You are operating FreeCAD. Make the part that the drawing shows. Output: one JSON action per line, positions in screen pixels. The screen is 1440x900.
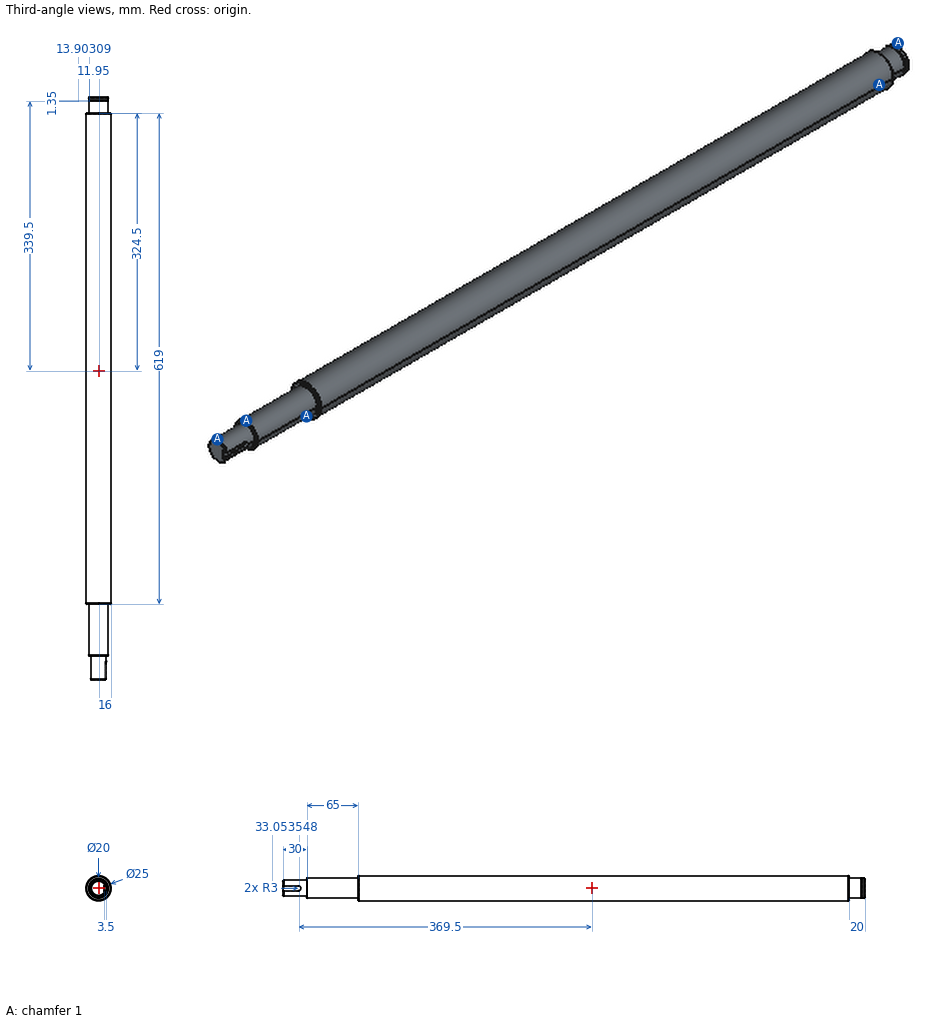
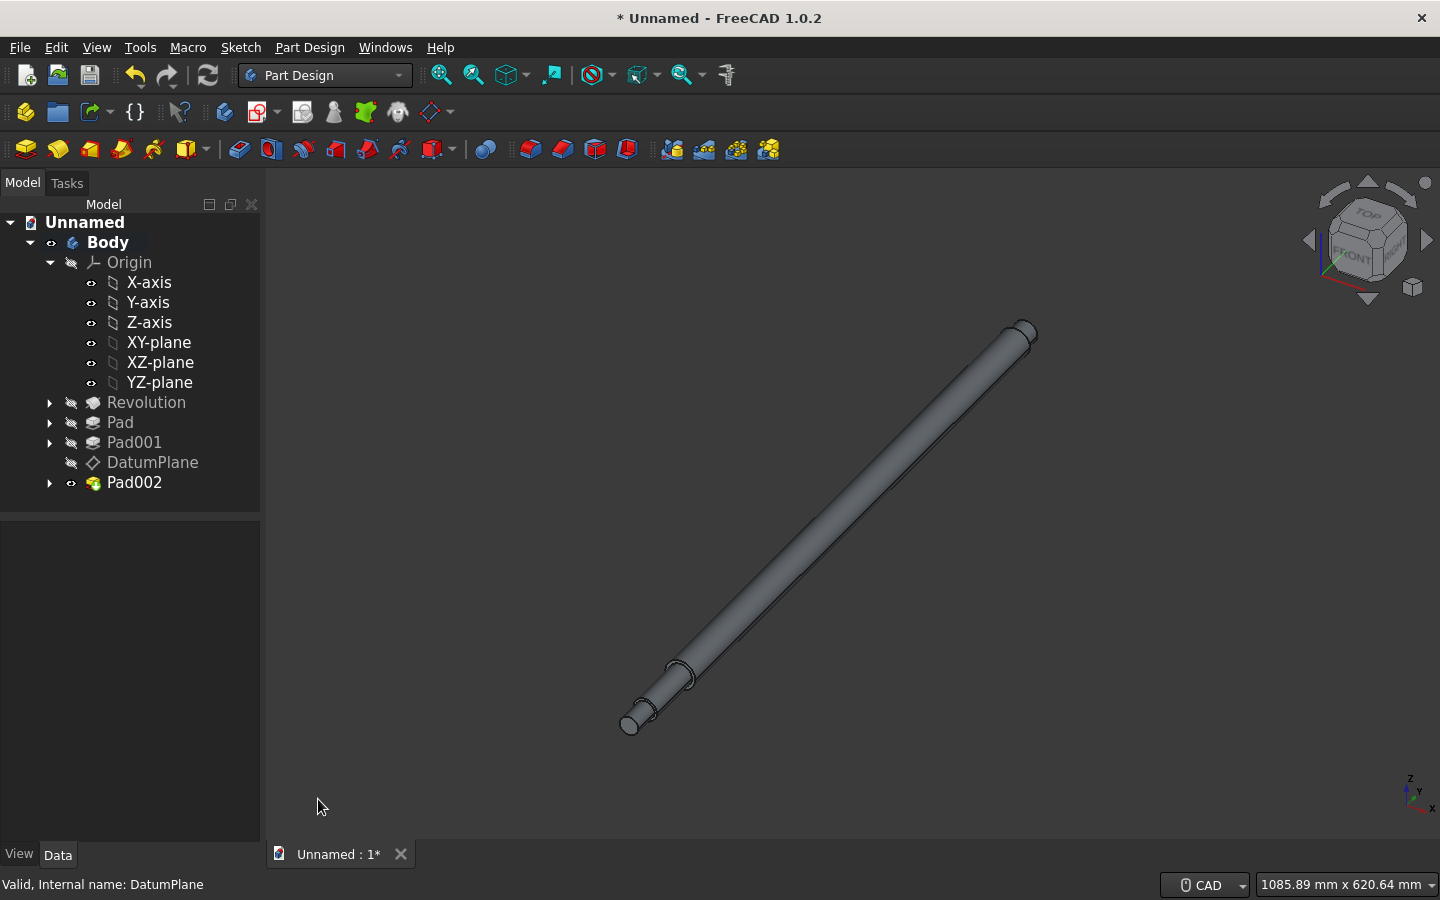
{"action": "left_click", "coordinate": [258, 112]}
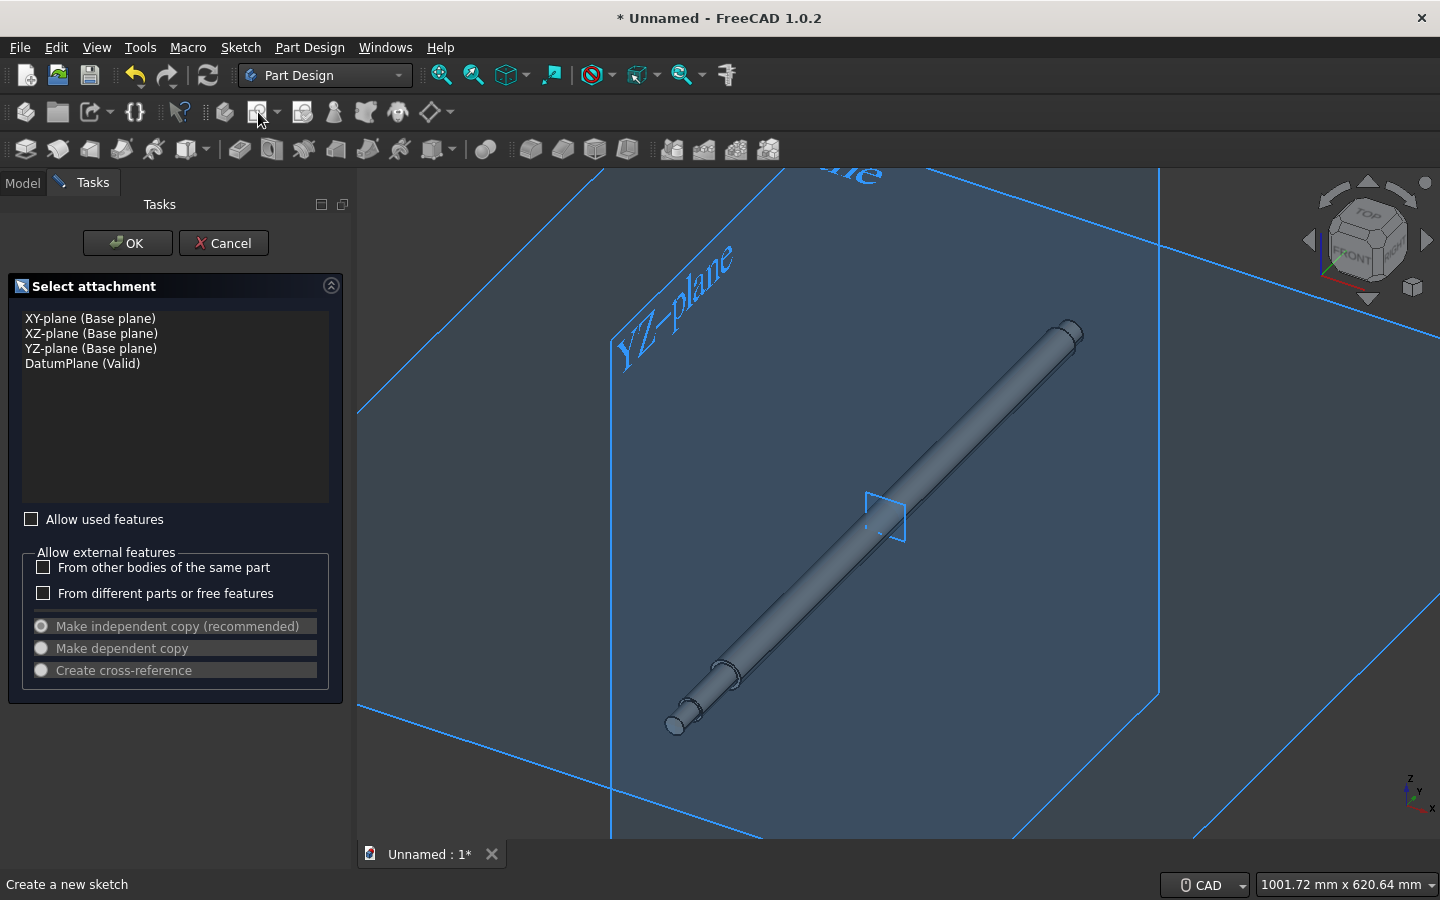
{"action": "left_click", "coordinate": [82, 318]}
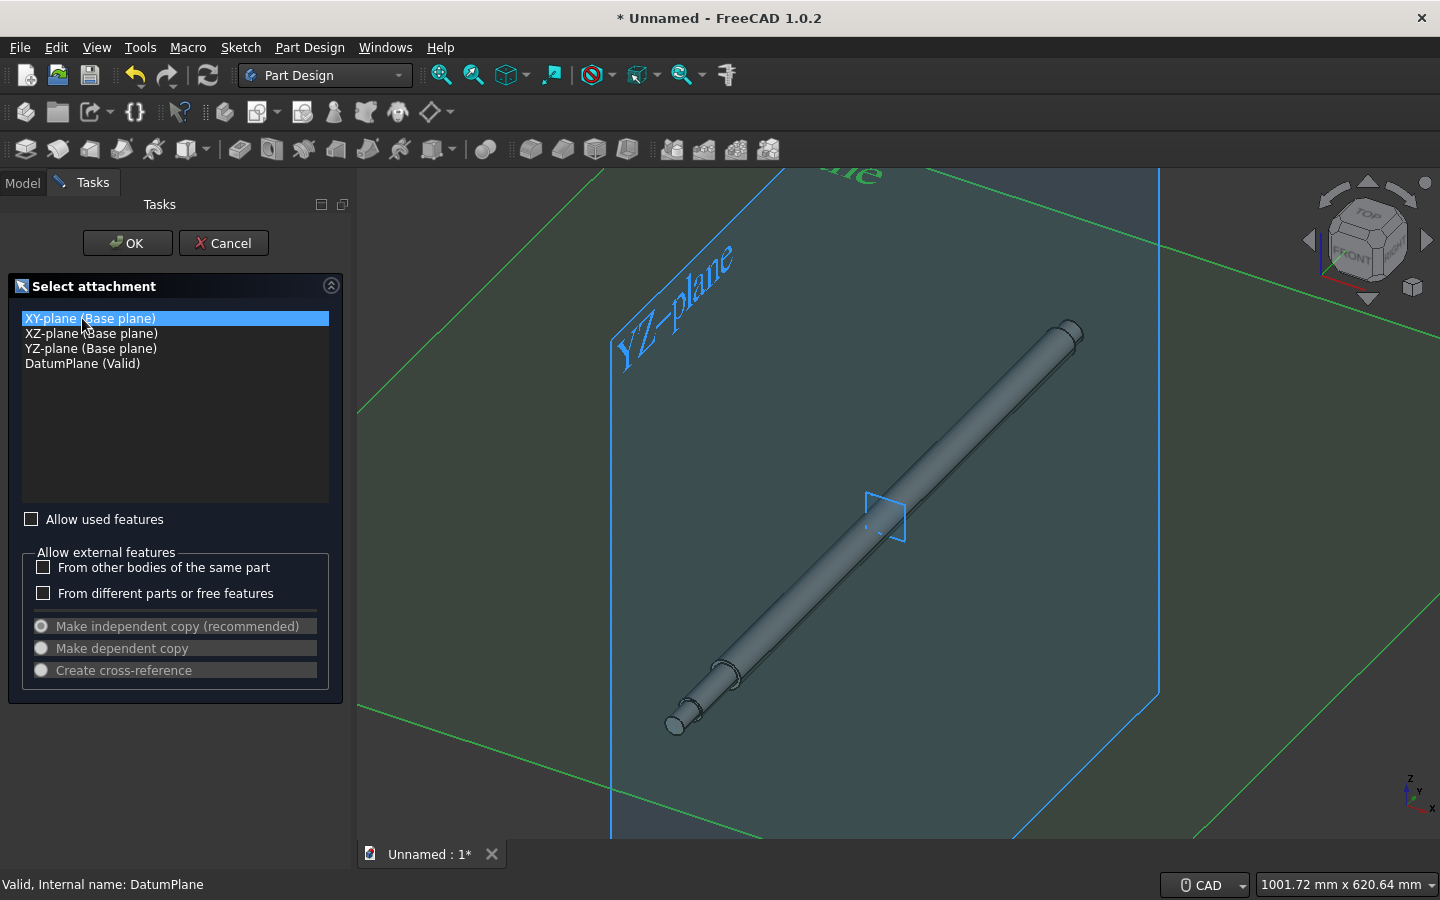
{"action": "left_click", "coordinate": [128, 243]}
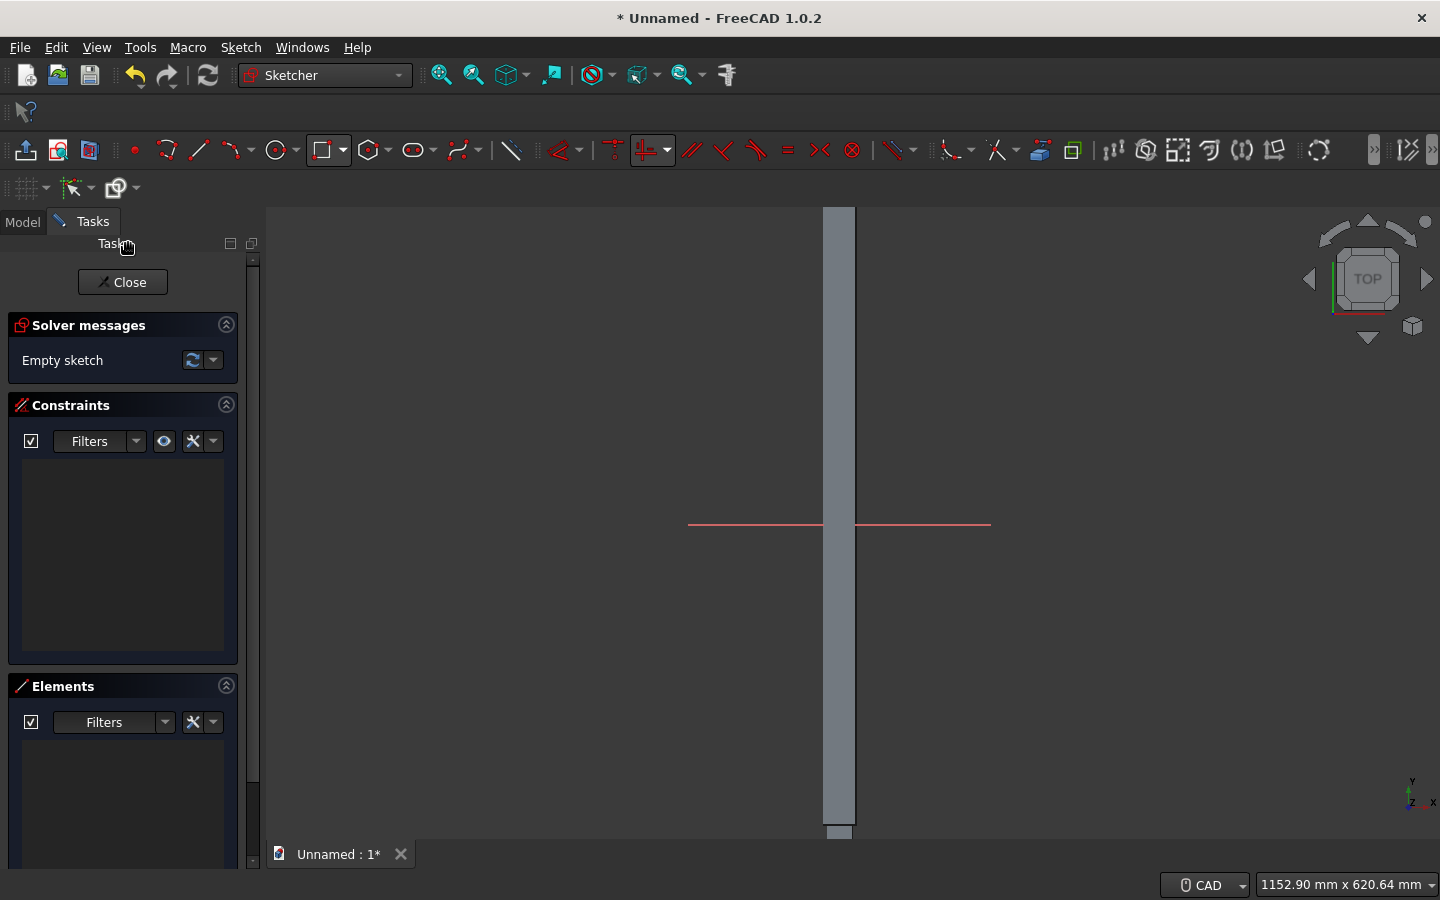
{"action": "left_click", "coordinate": [90, 150]}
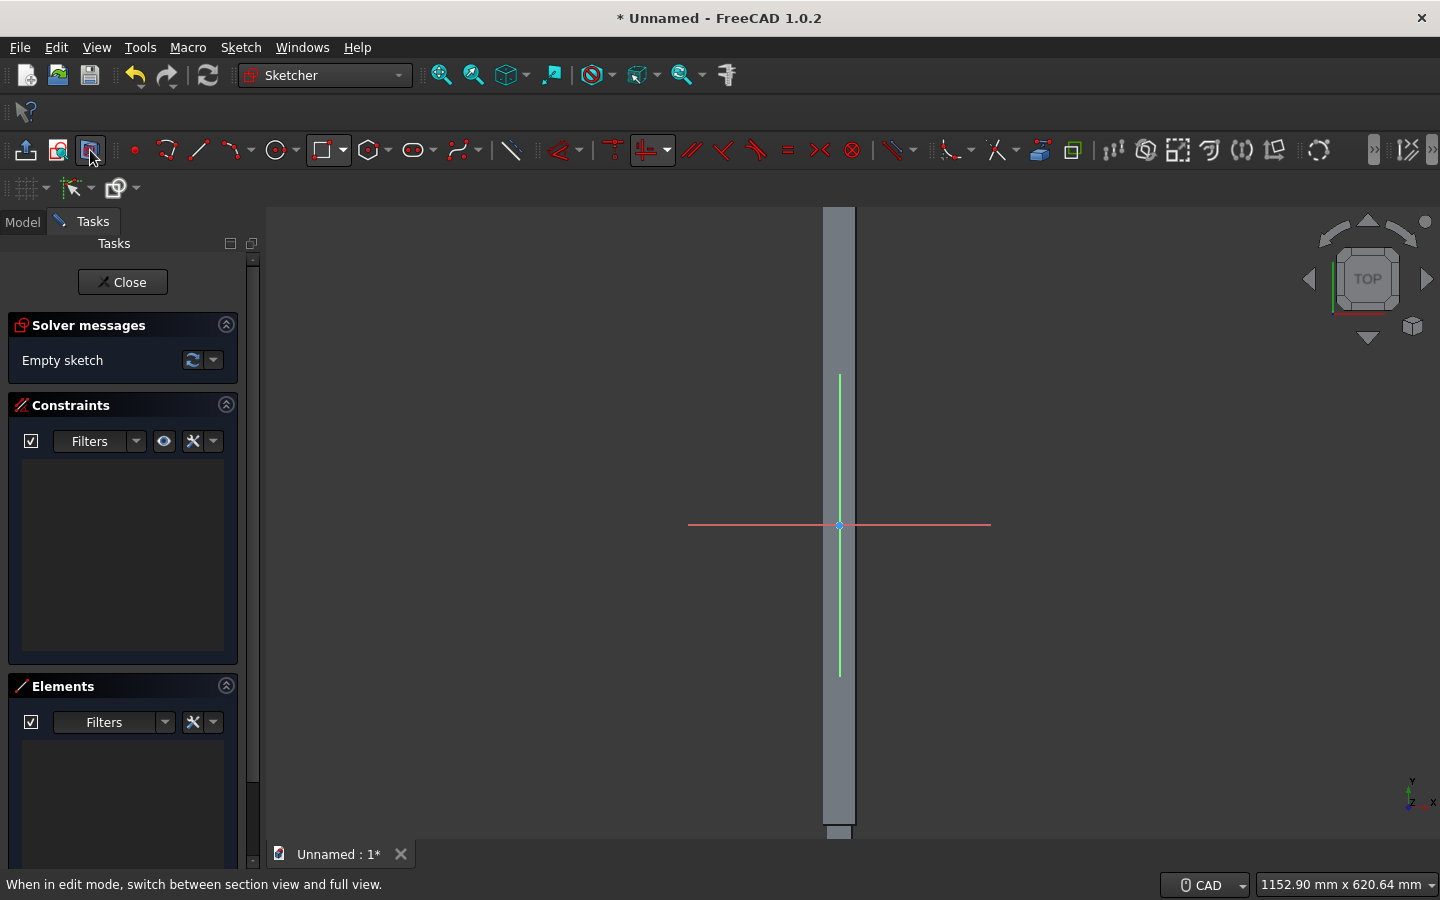
{"action": "scroll", "coordinate": [784, 523], "scroll_direction": "down", "scroll_amount": 5}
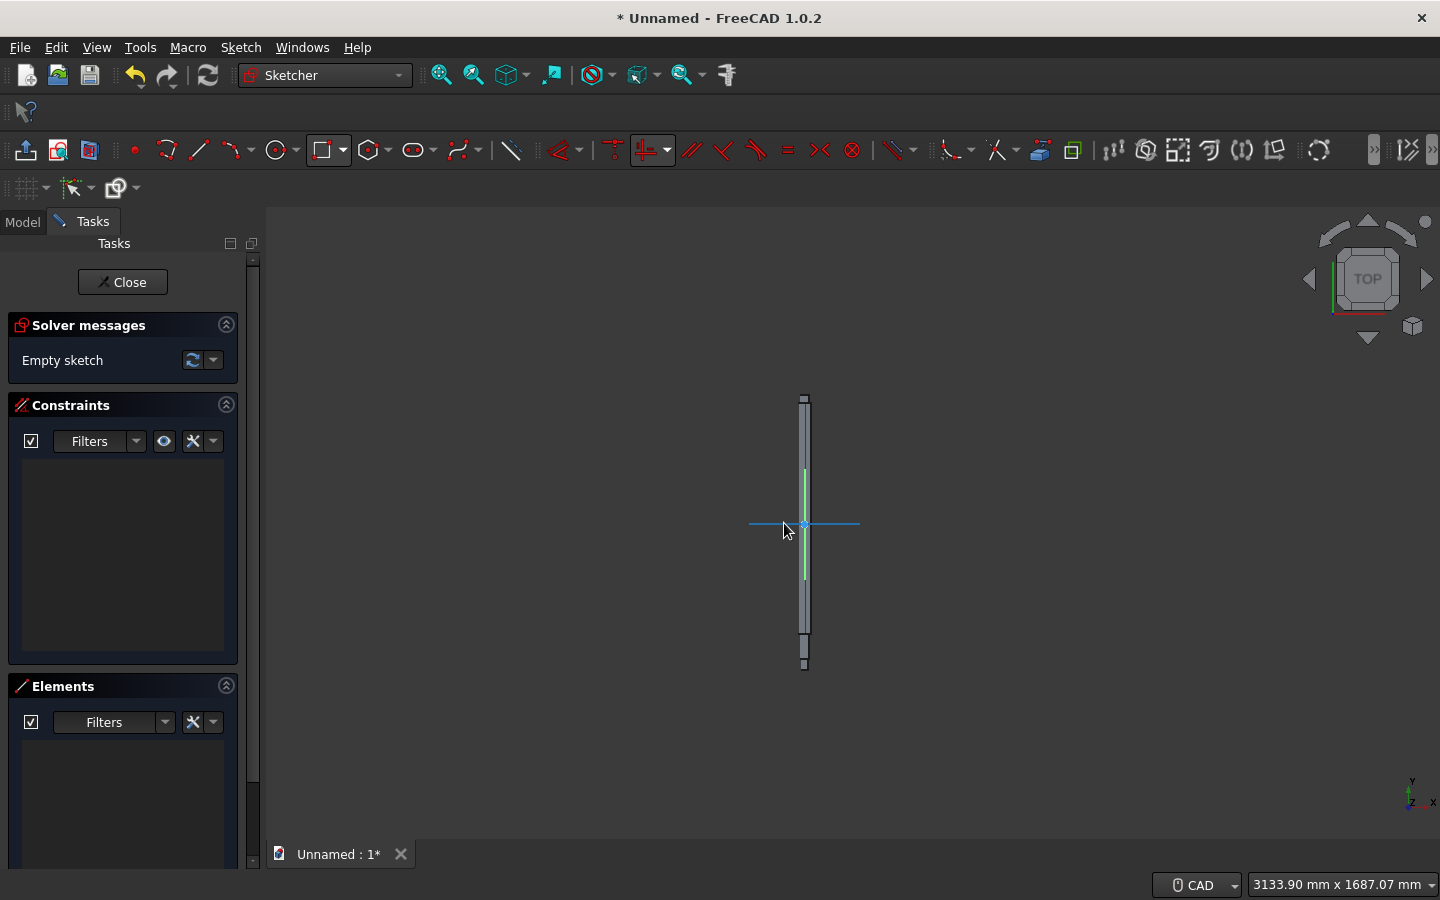
{"action": "scroll", "coordinate": [798, 390], "scroll_direction": "up", "scroll_amount": 15}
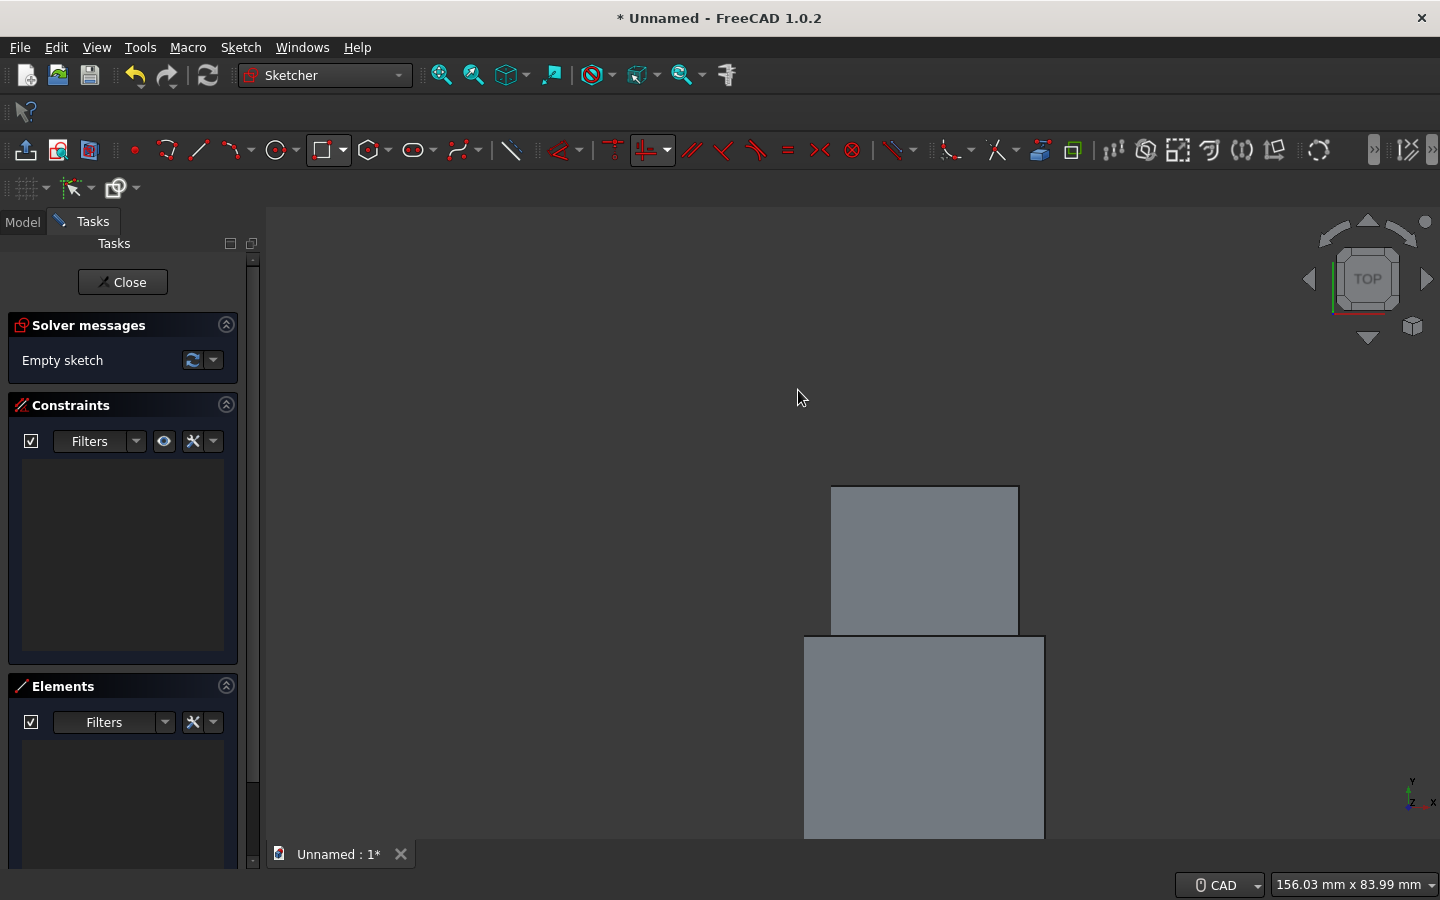
{"action": "scroll", "coordinate": [782, 518], "scroll_direction": "up", "scroll_amount": 9}